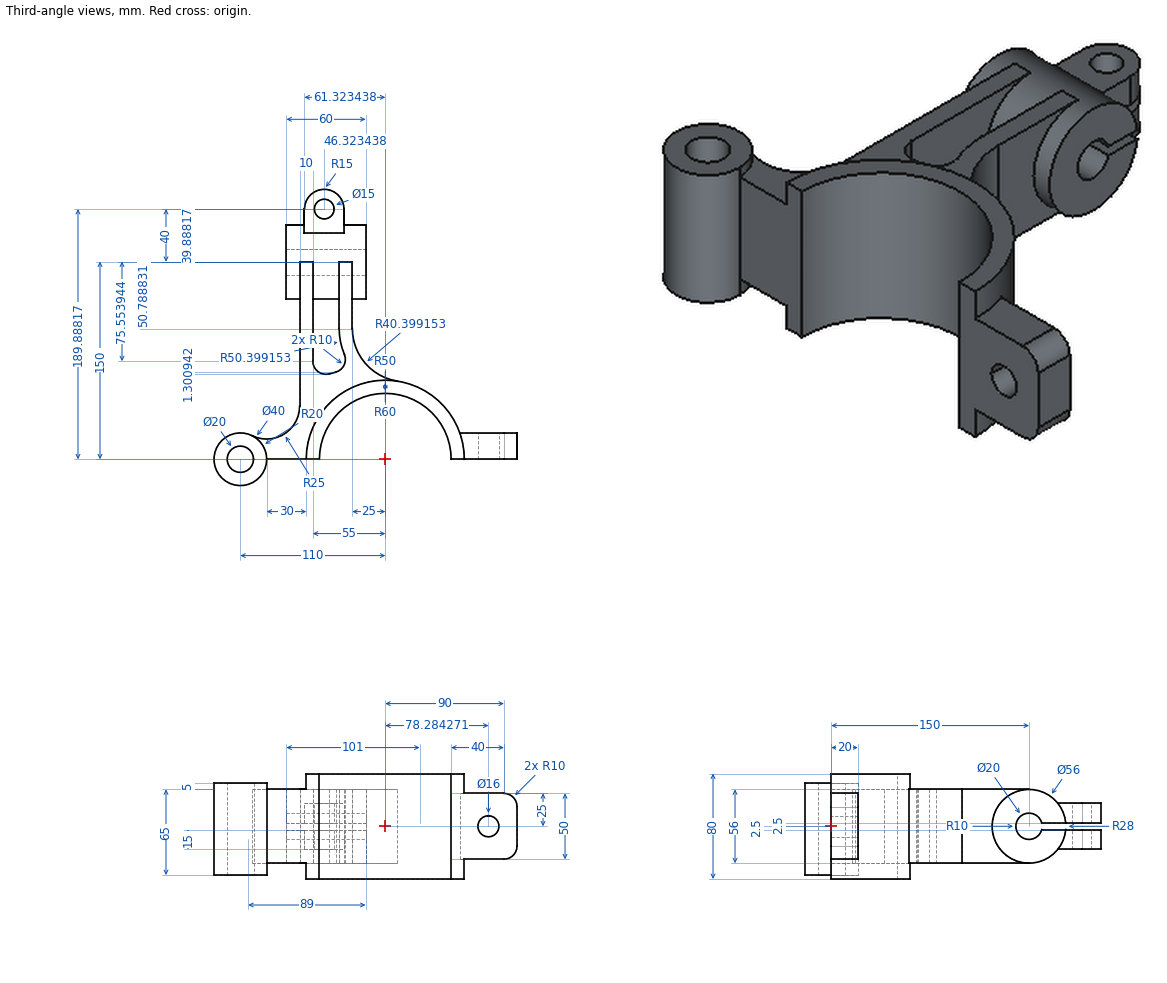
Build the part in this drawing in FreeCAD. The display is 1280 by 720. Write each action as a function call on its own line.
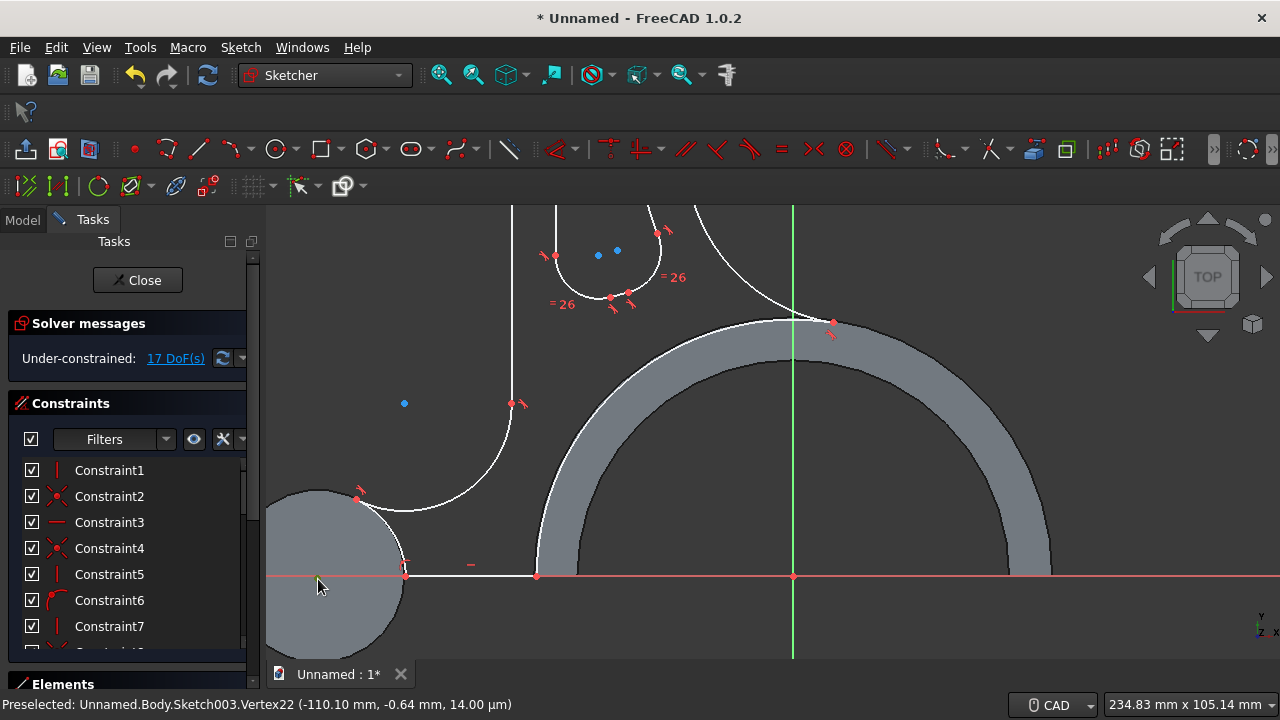
click(353, 576)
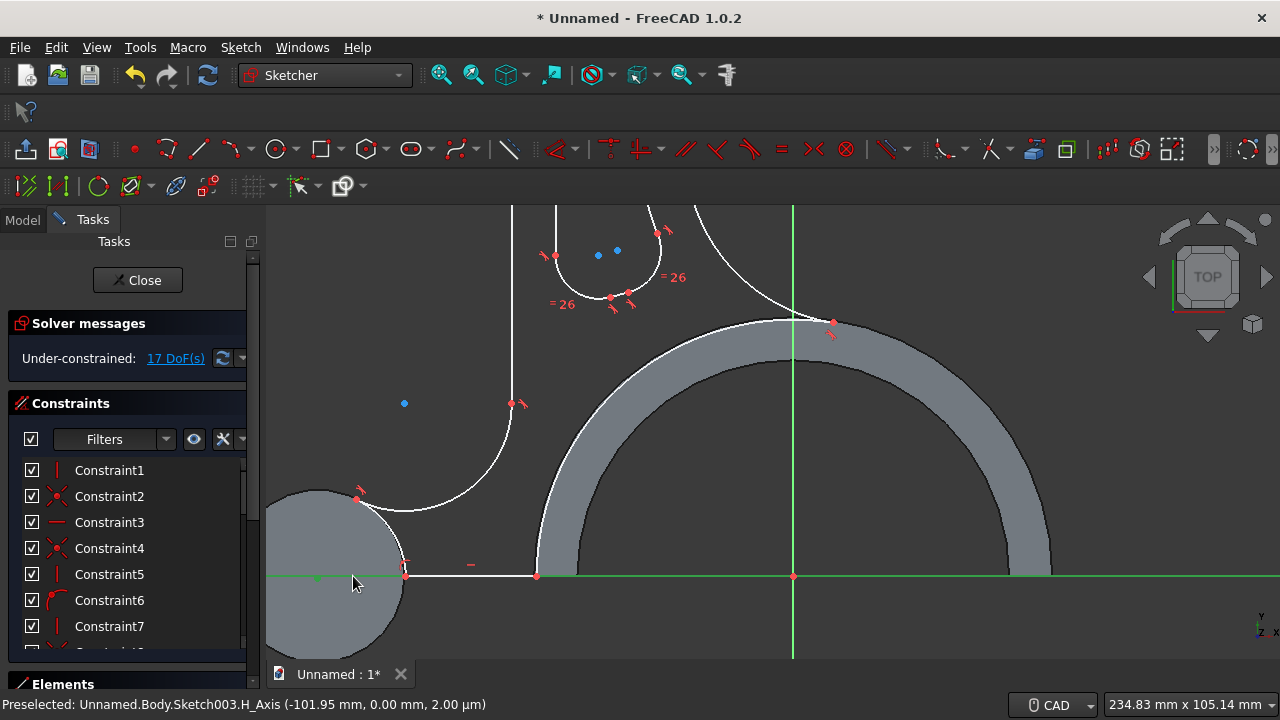
key(c)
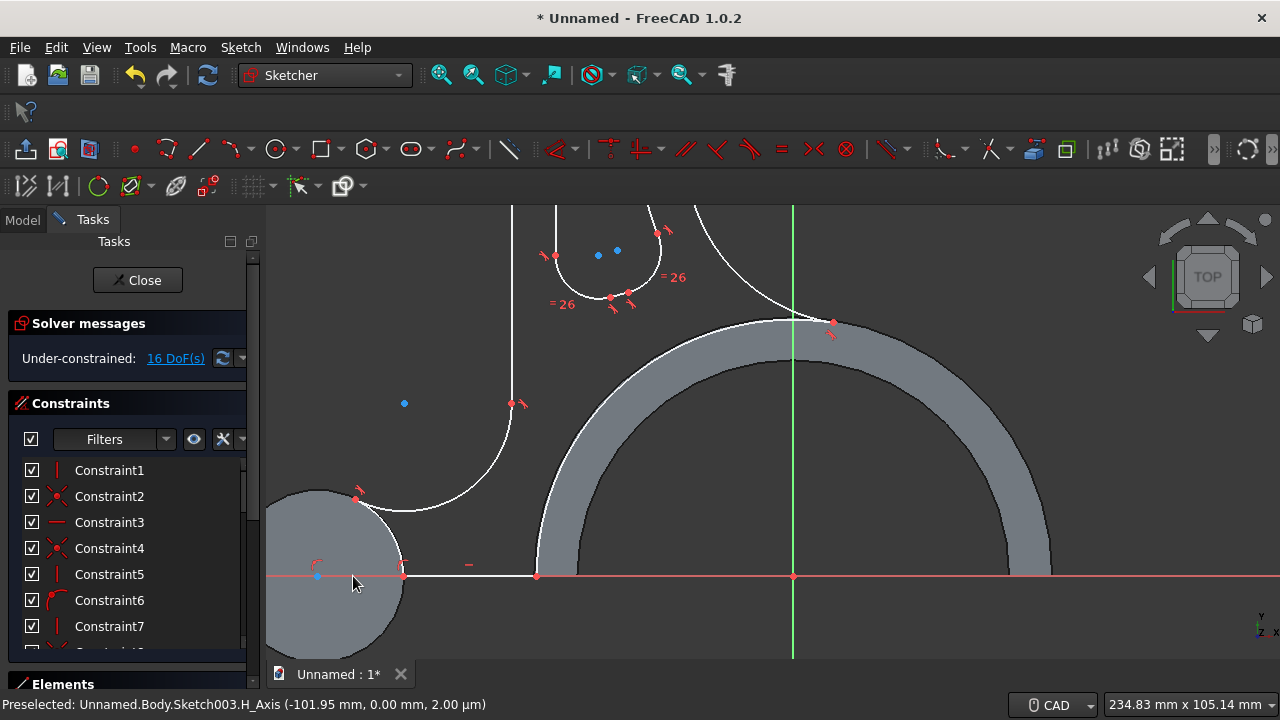
key(d)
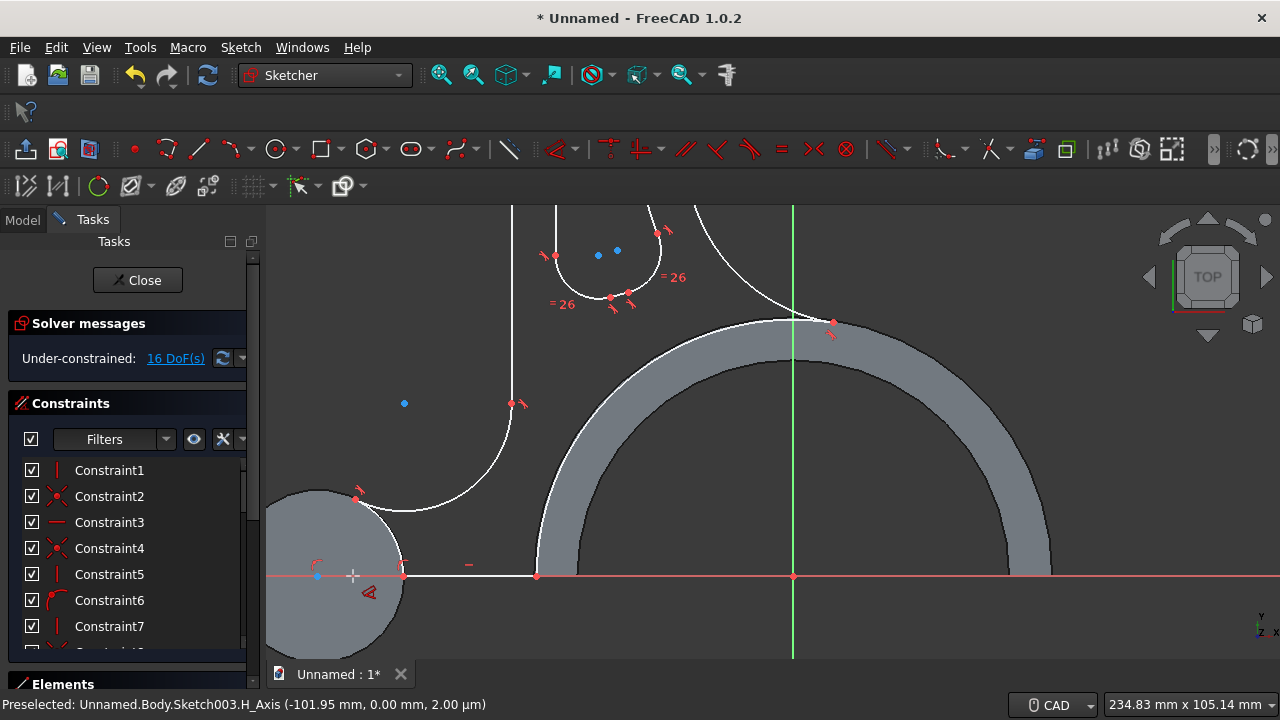
click(420, 510)
click(425, 542)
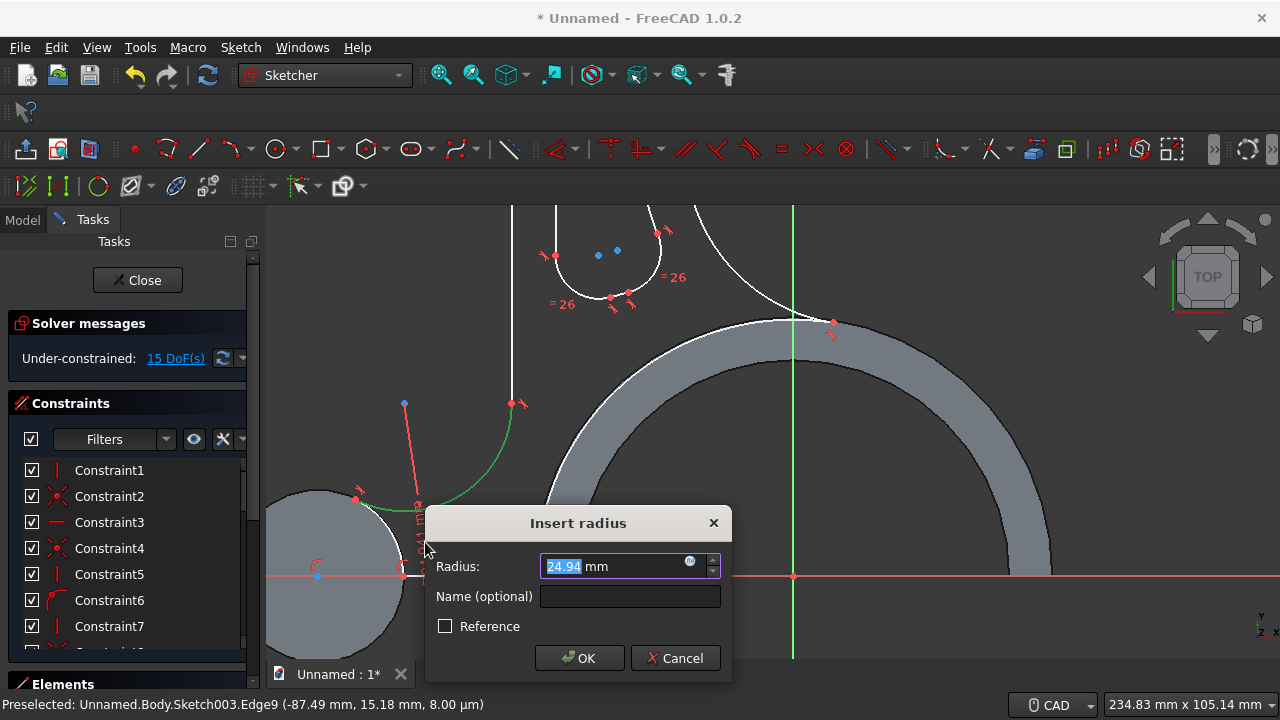
text(25)
key(Return)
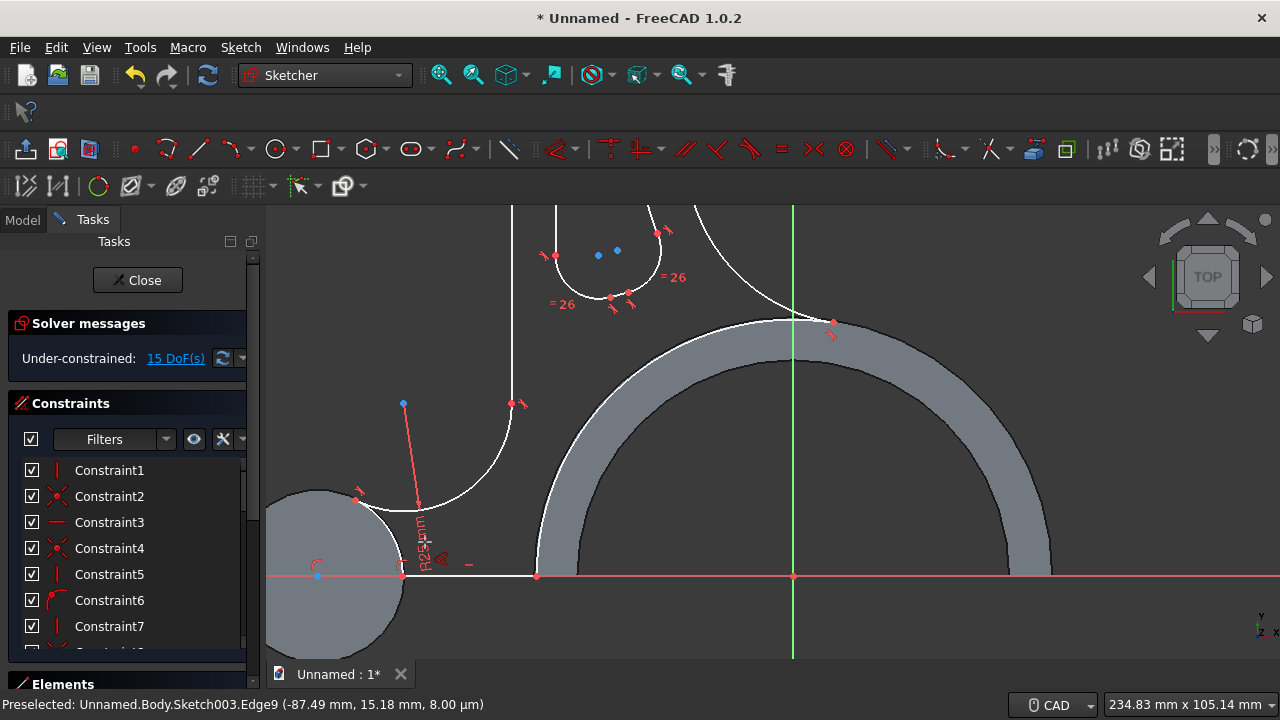
click(398, 548)
click(433, 595)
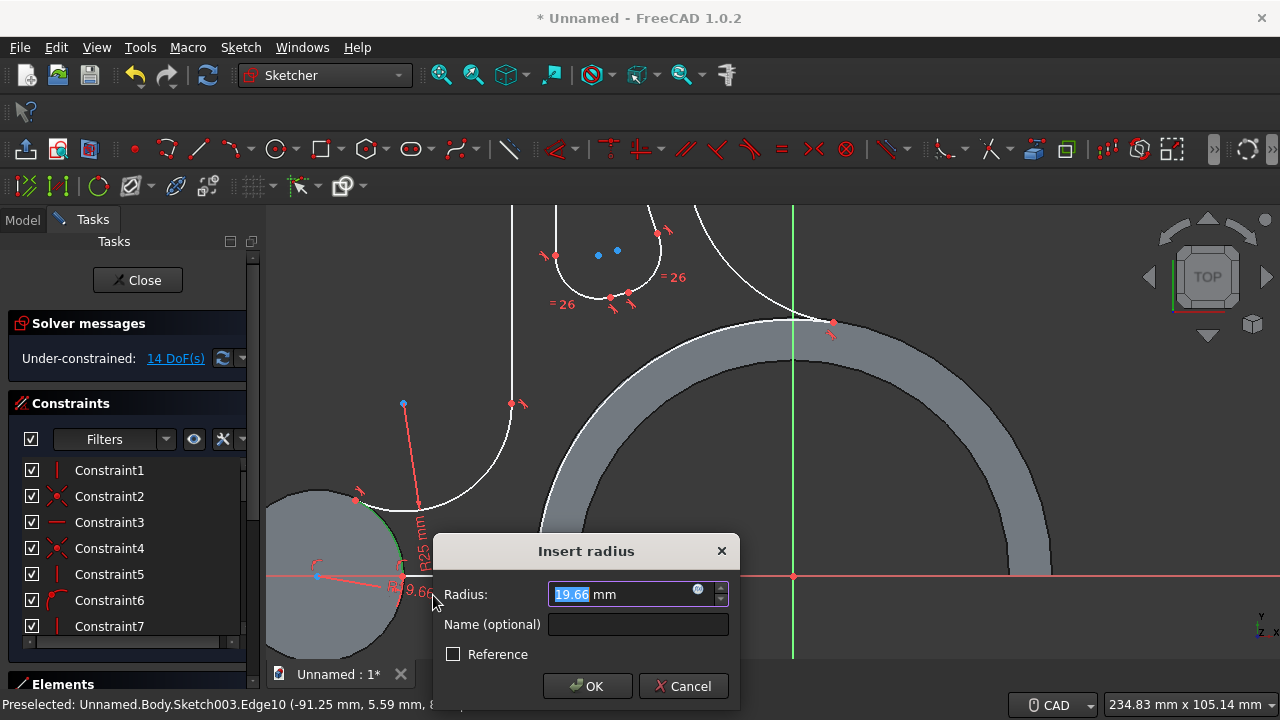
text(20)
key(Return)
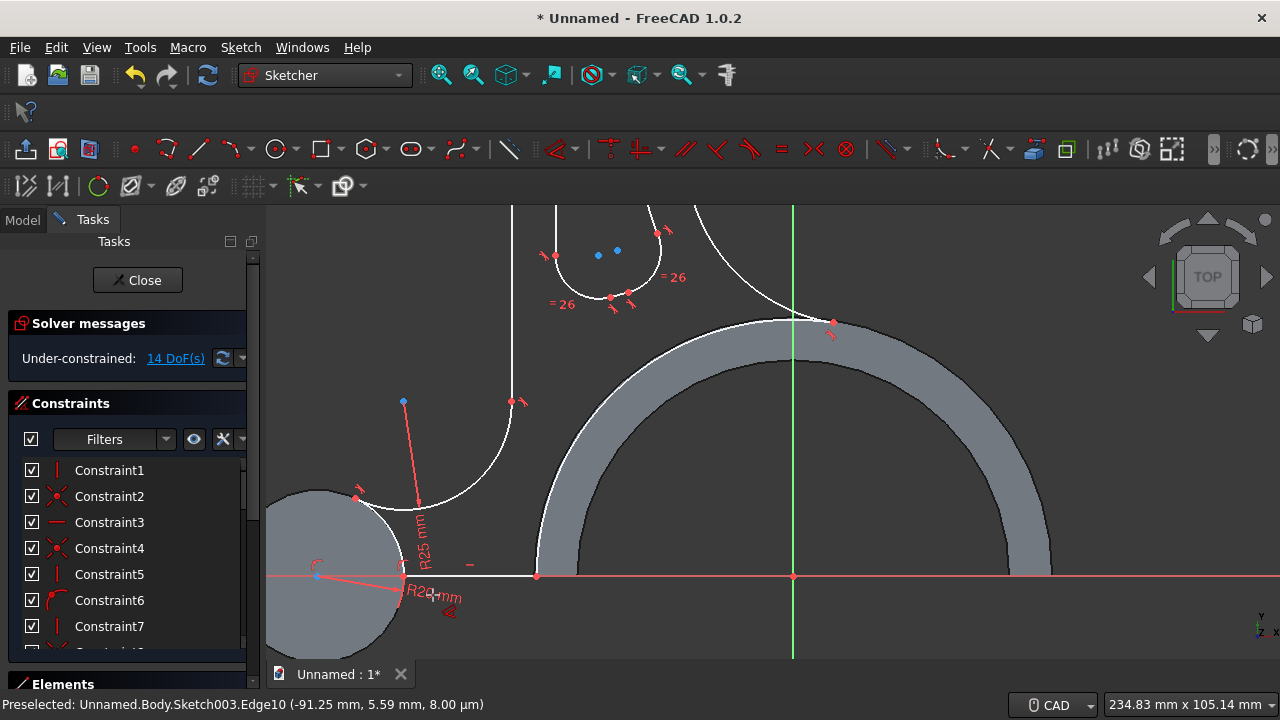
click(703, 336)
click(692, 306)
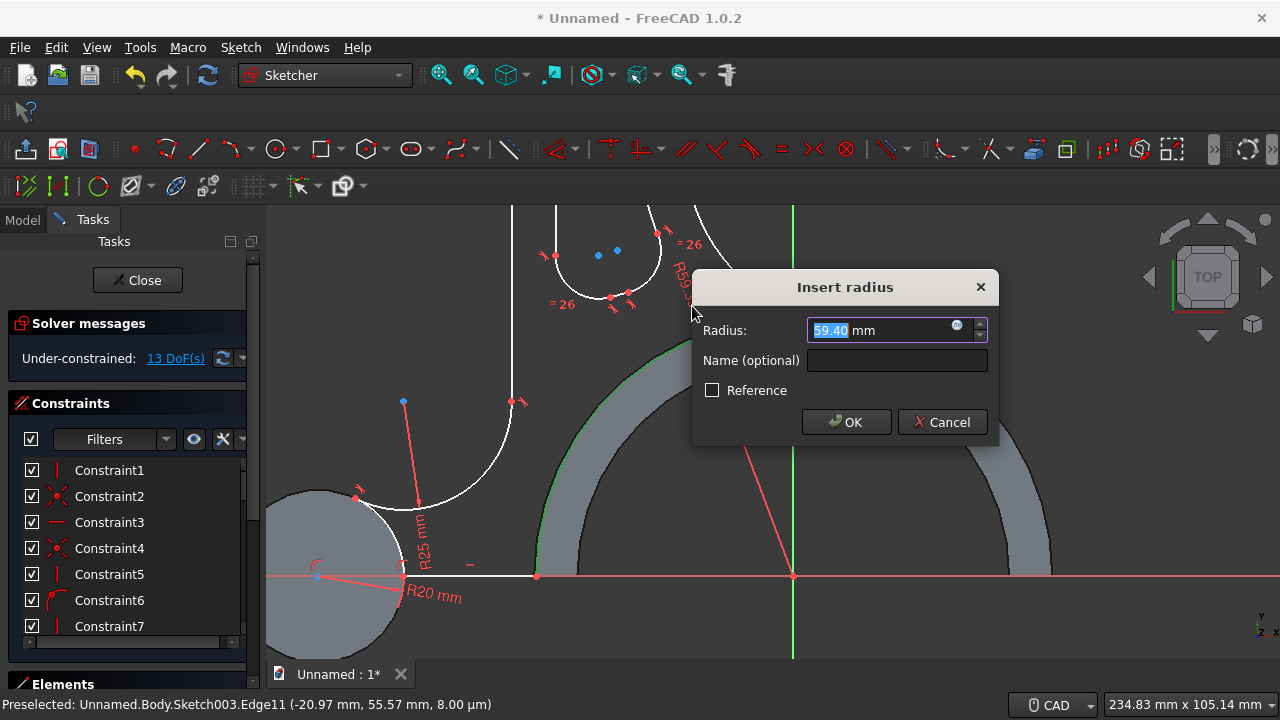
text(60)
key(Return)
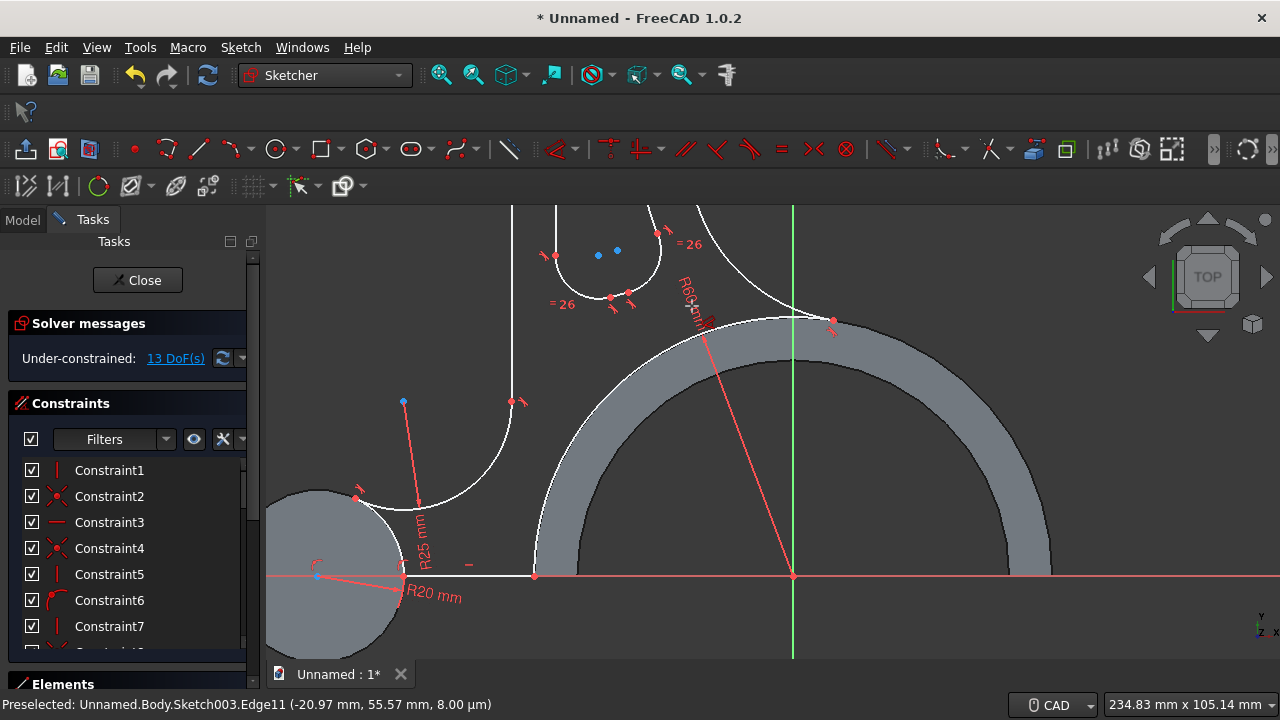
click(766, 294)
click(680, 246)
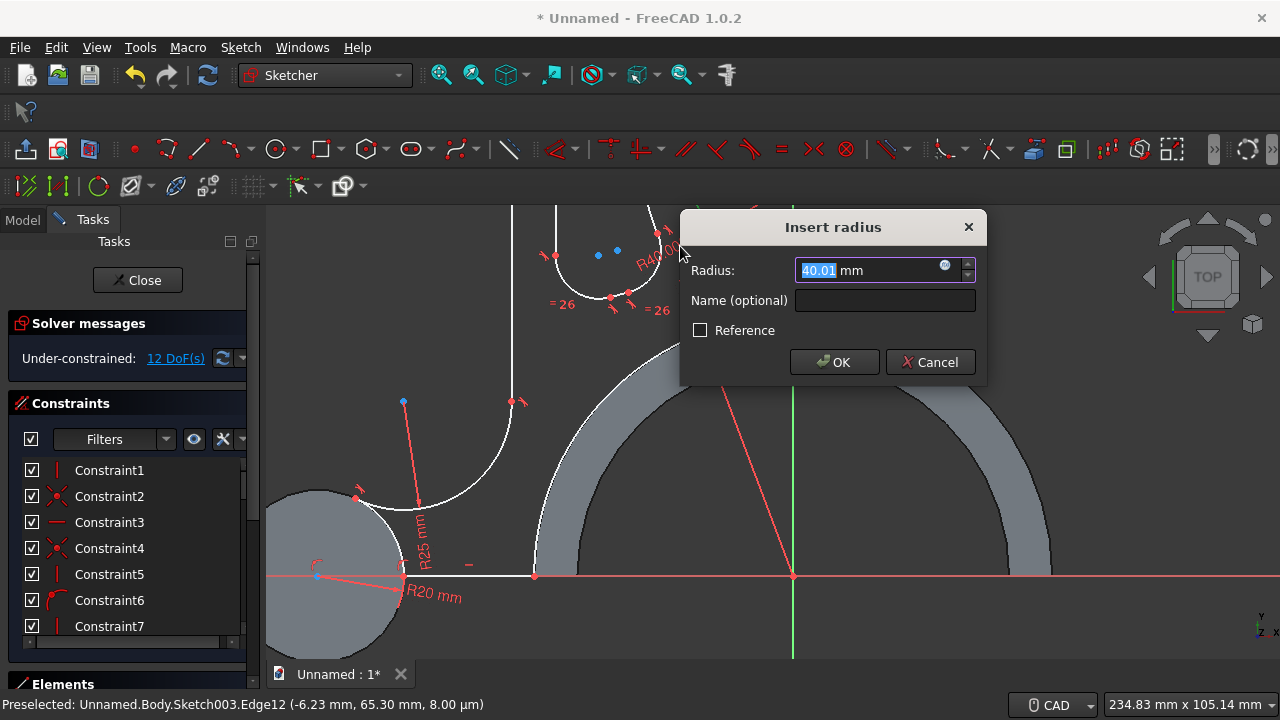
text(40.399153)
key(Return)